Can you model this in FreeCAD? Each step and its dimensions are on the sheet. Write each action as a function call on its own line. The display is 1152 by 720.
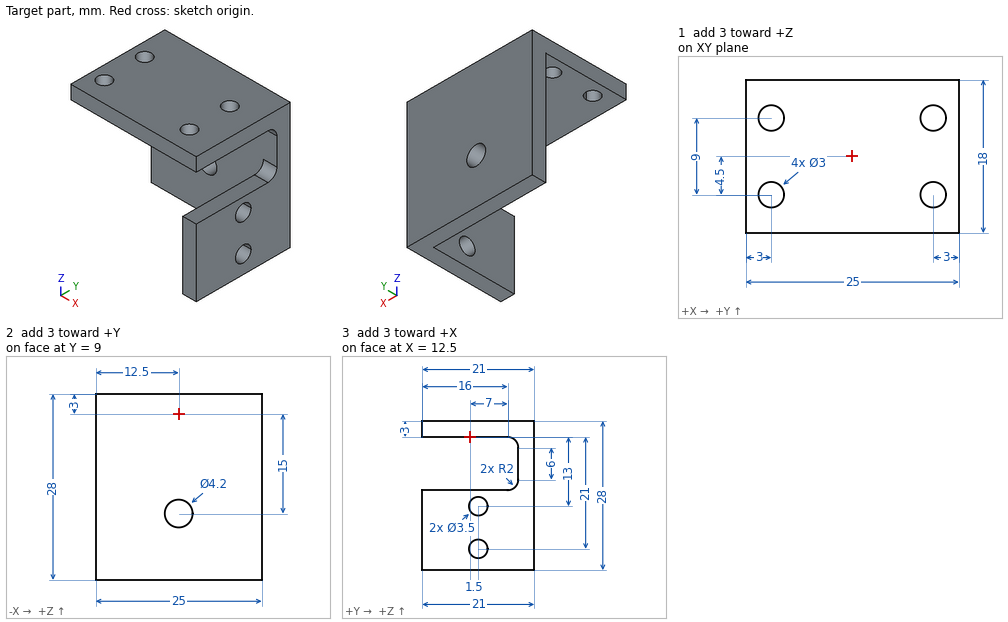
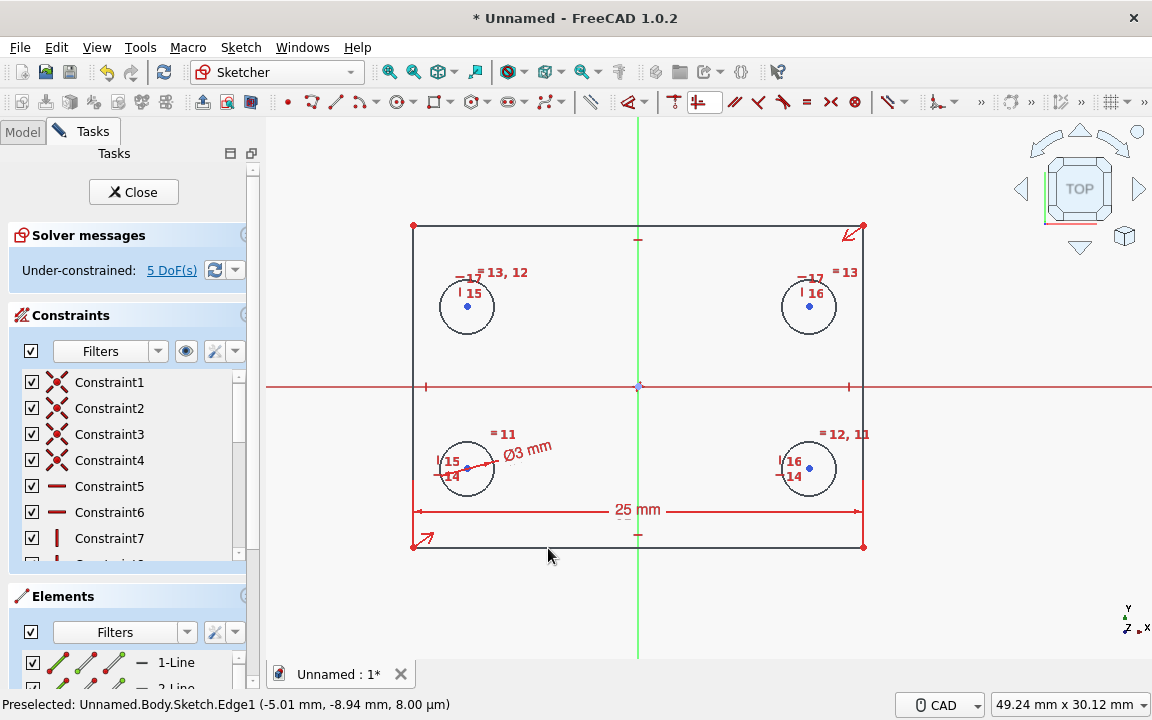
click(863, 451)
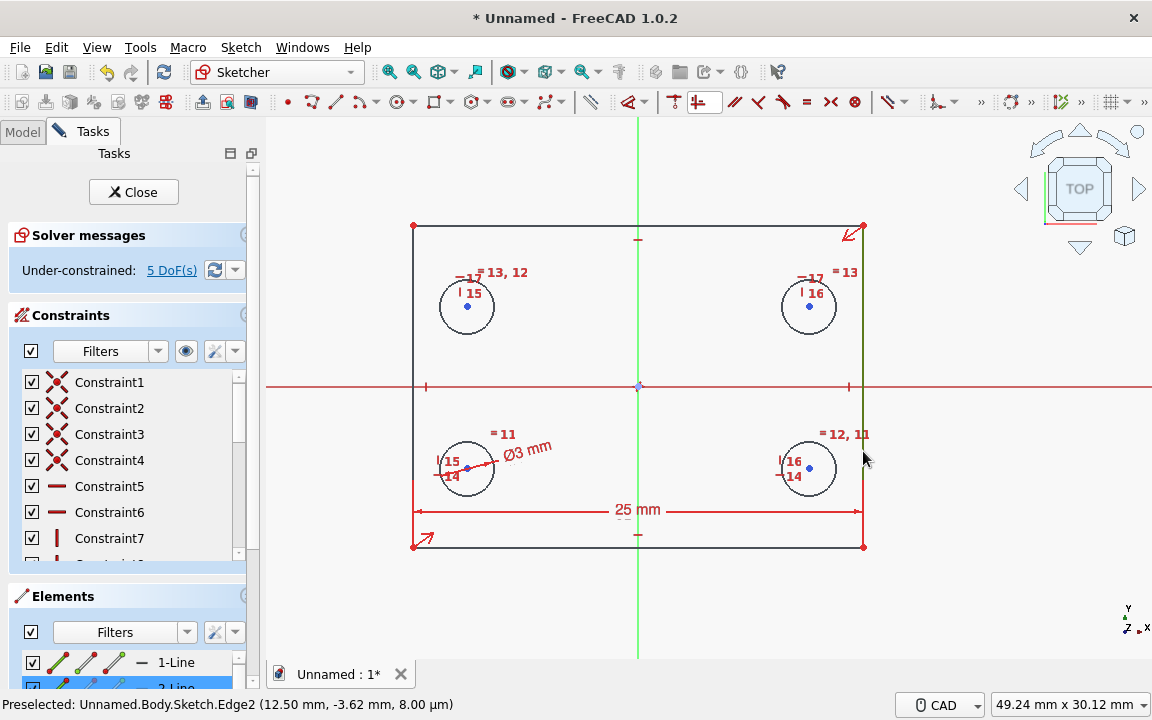
key(i)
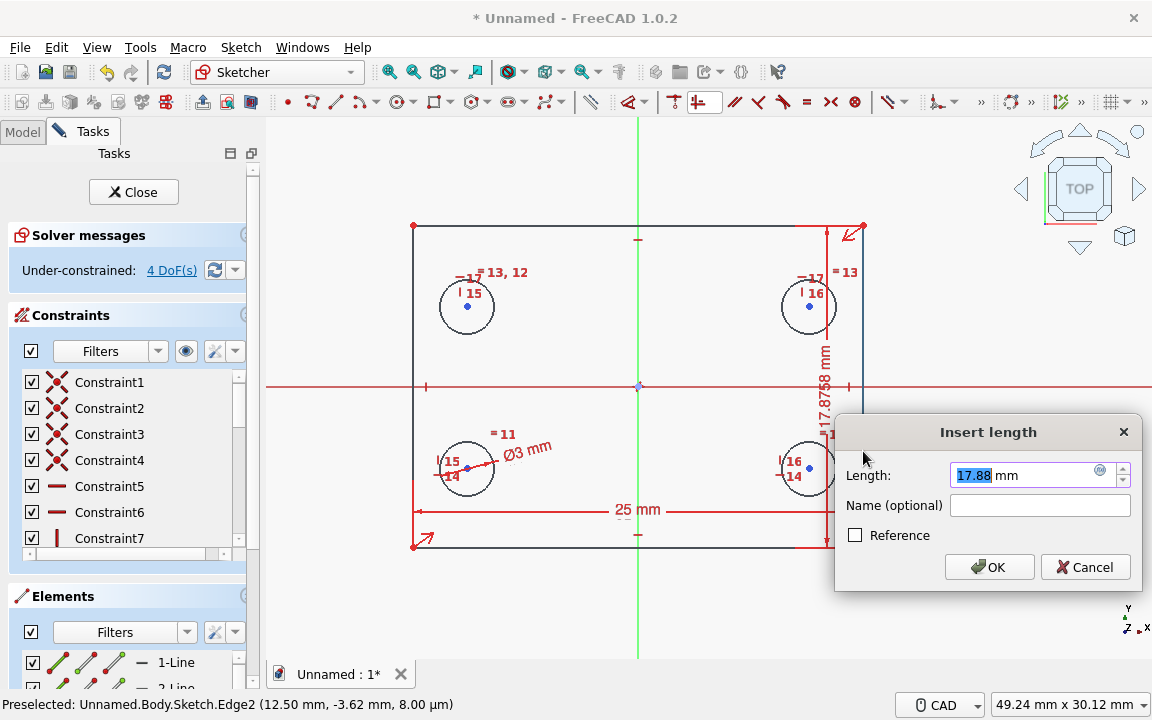
text(18)
key(Return)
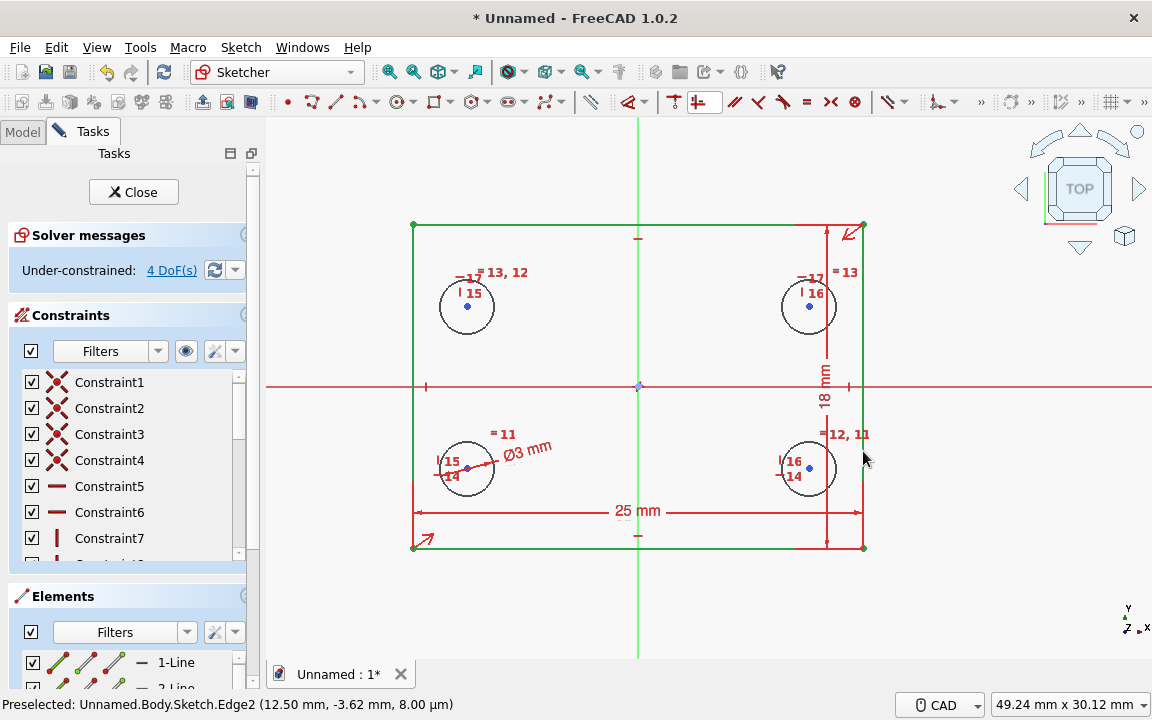
click(413, 549)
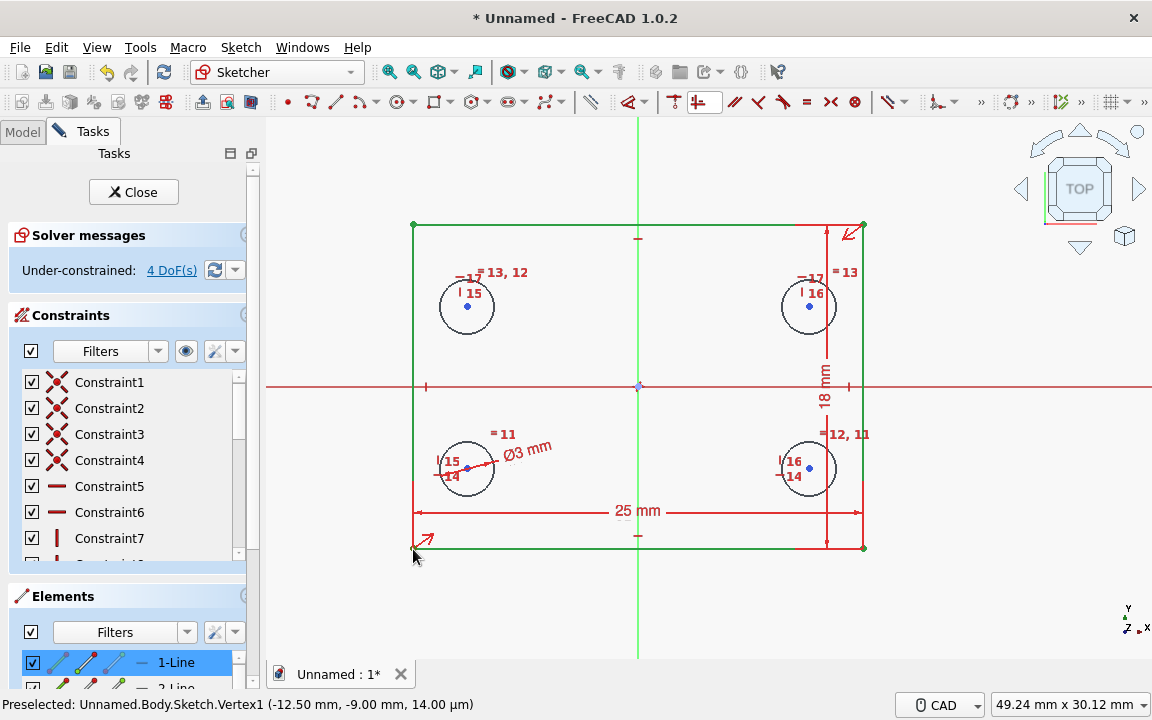
click(467, 469)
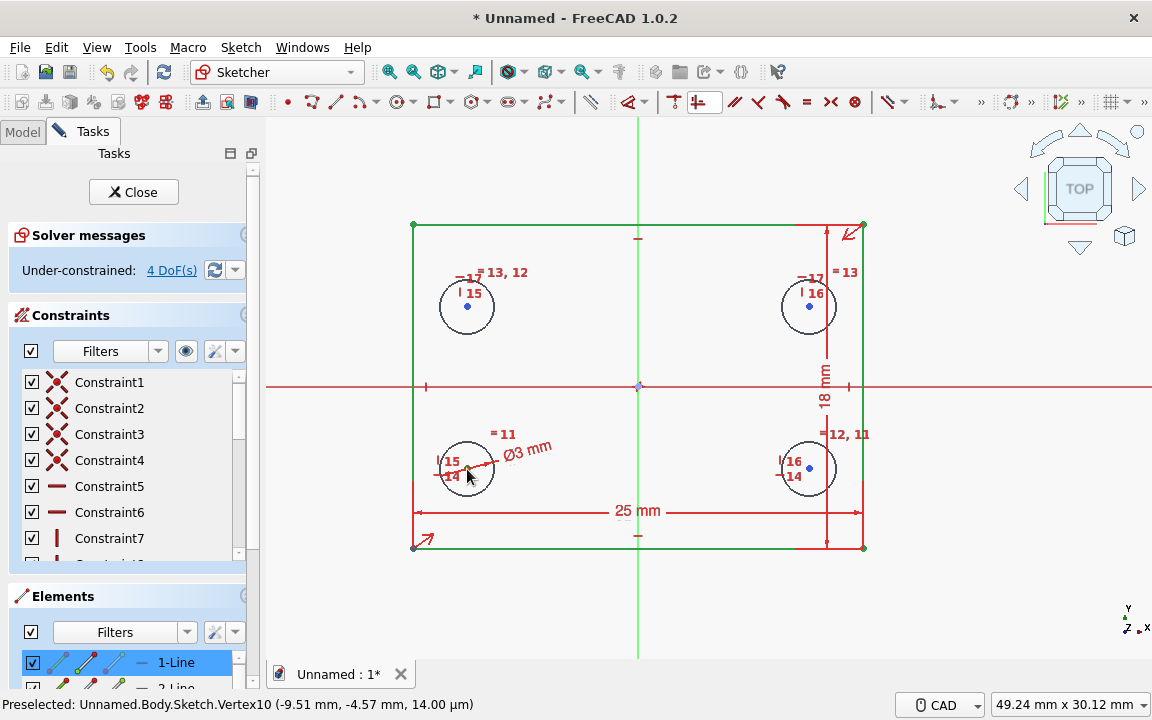
key(l)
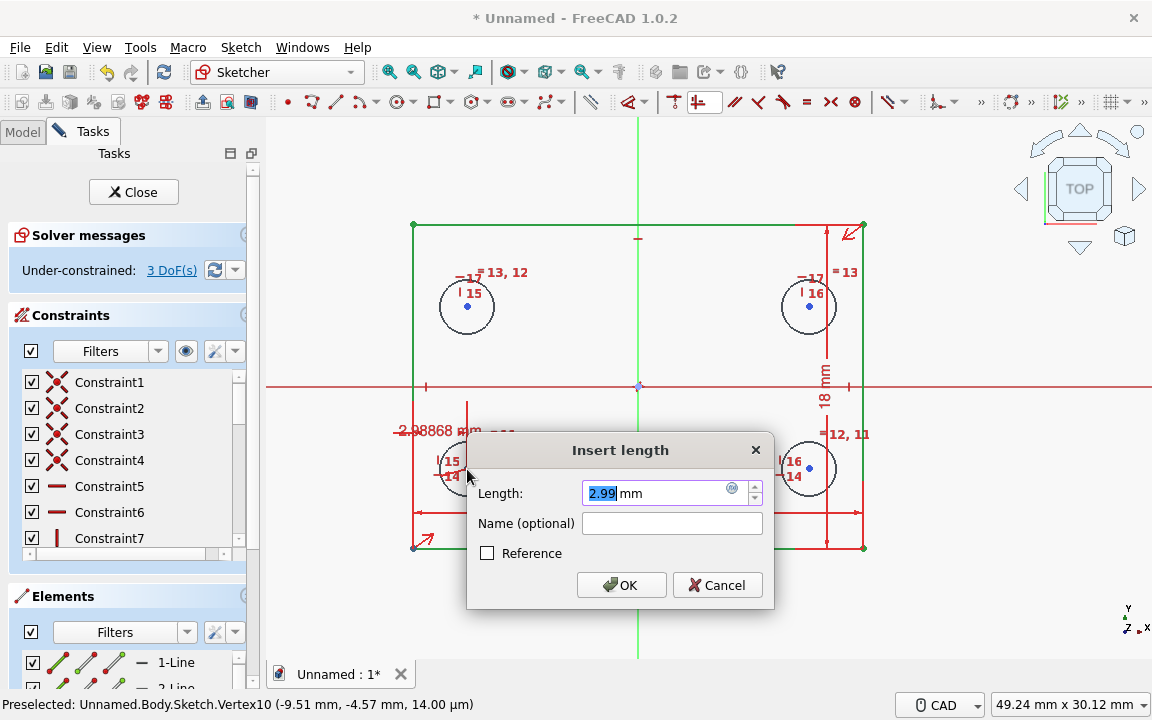
text(3)
key(Return)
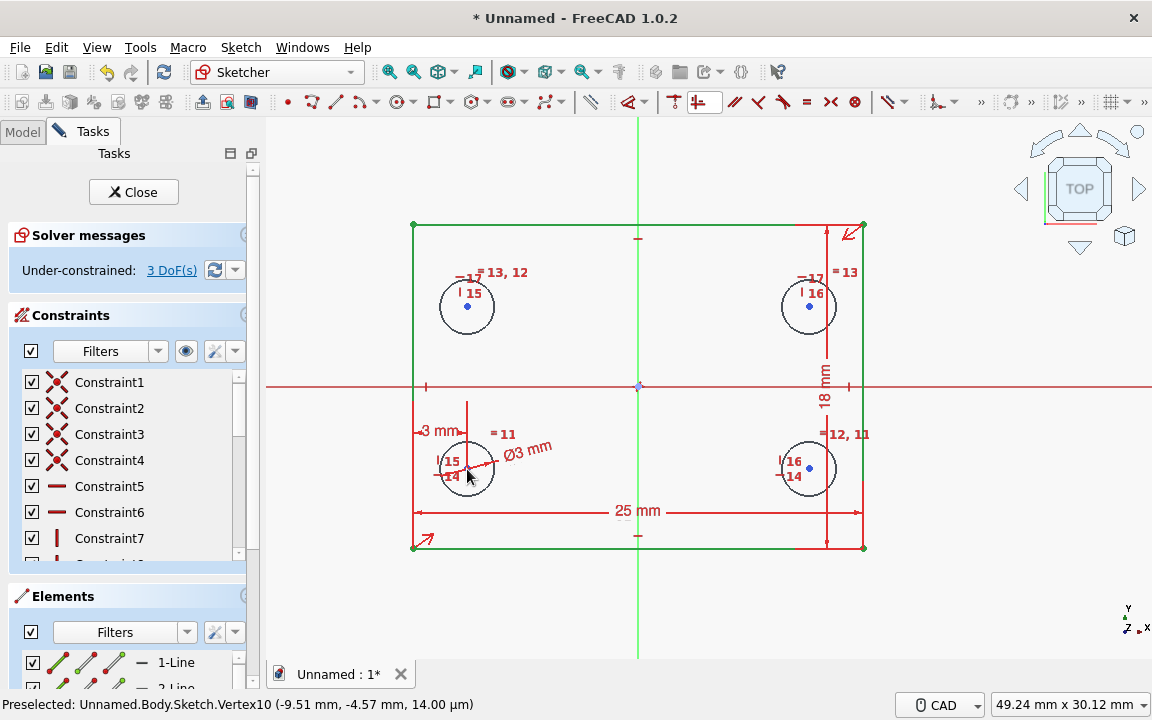
click(863, 549)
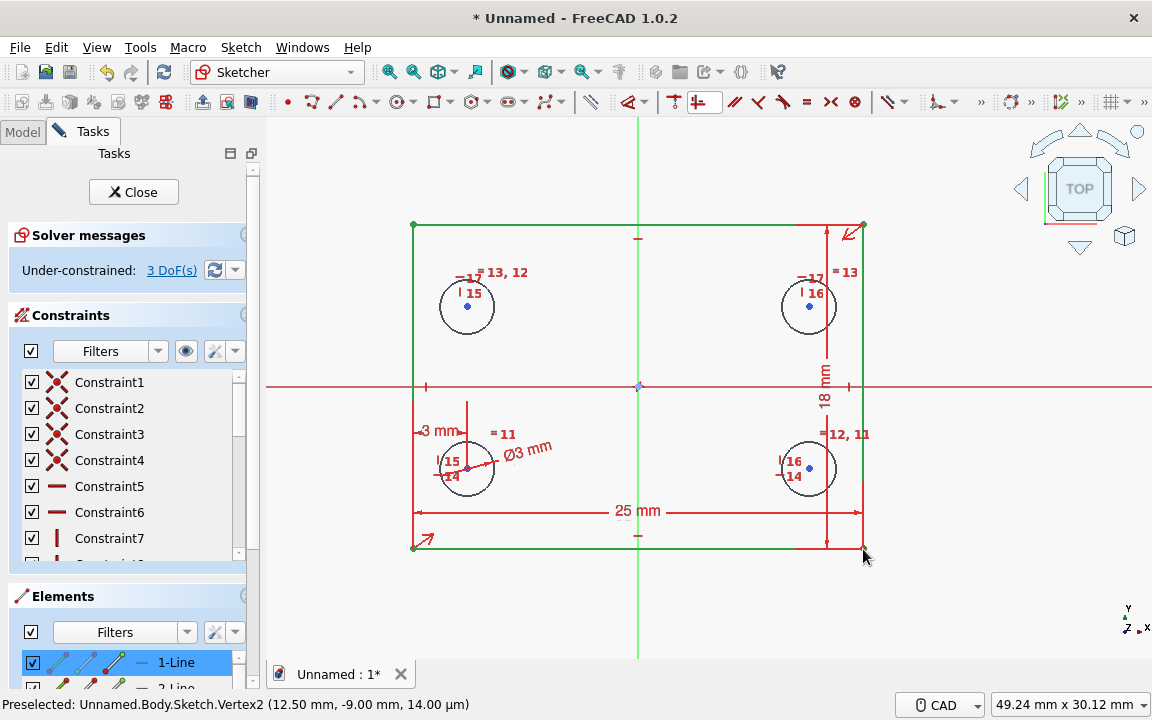
click(809, 469)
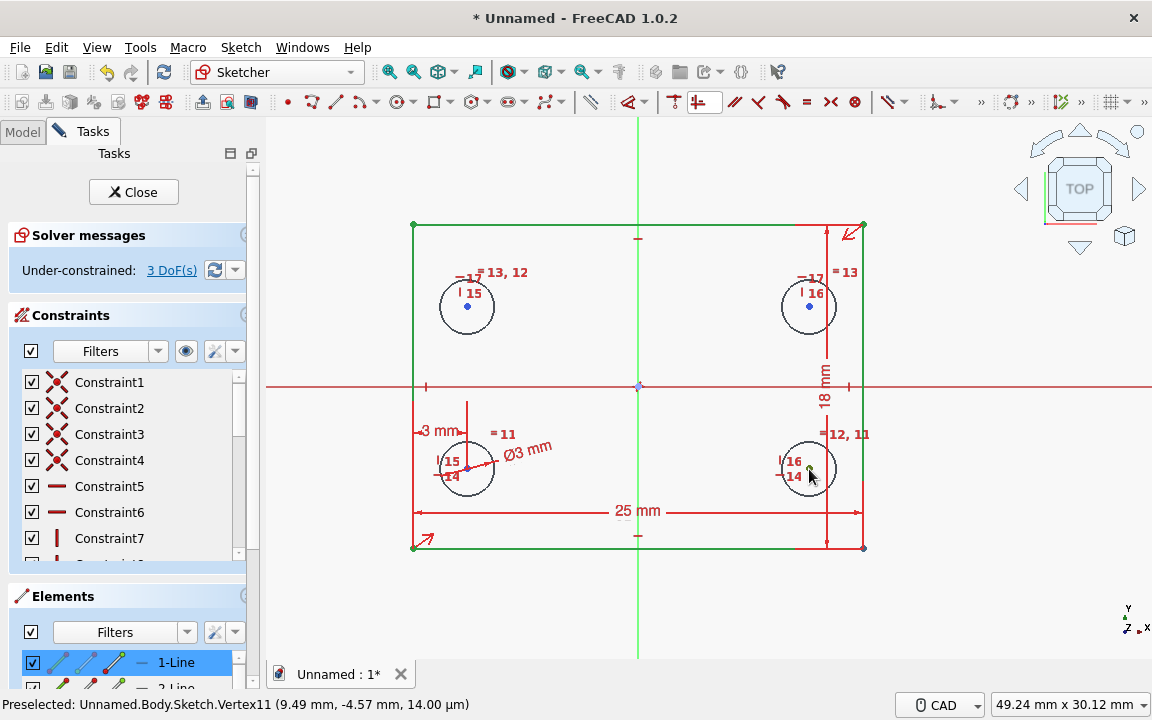
click(646, 102)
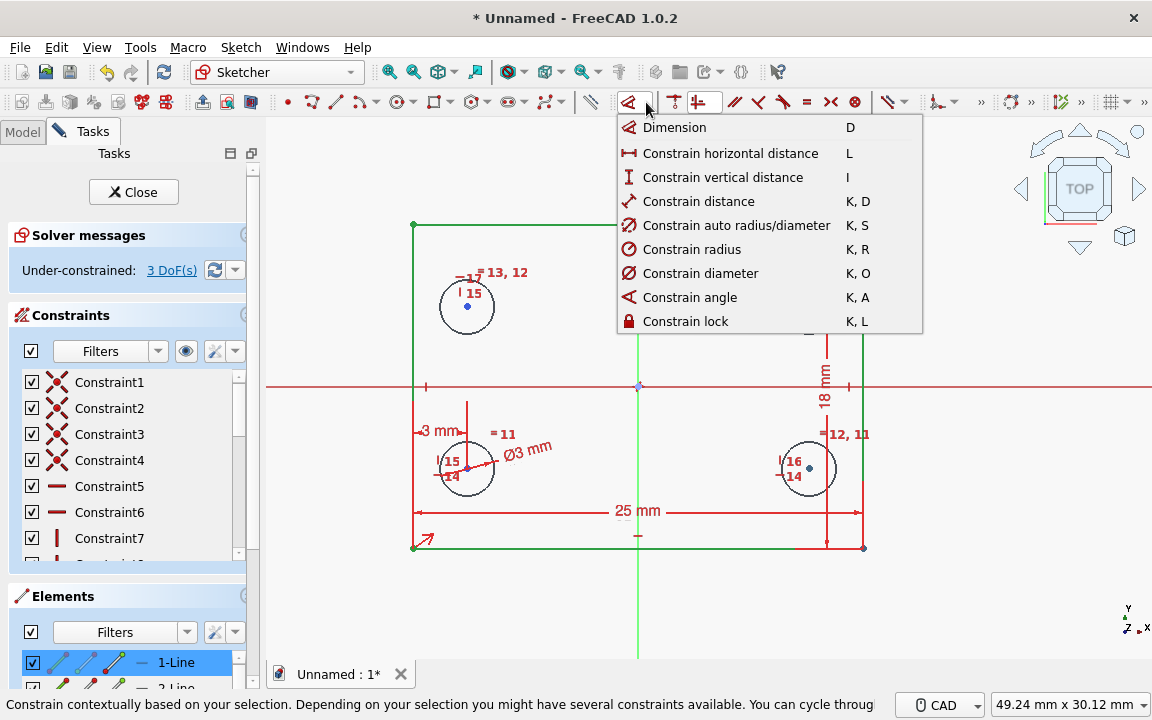
click(770, 153)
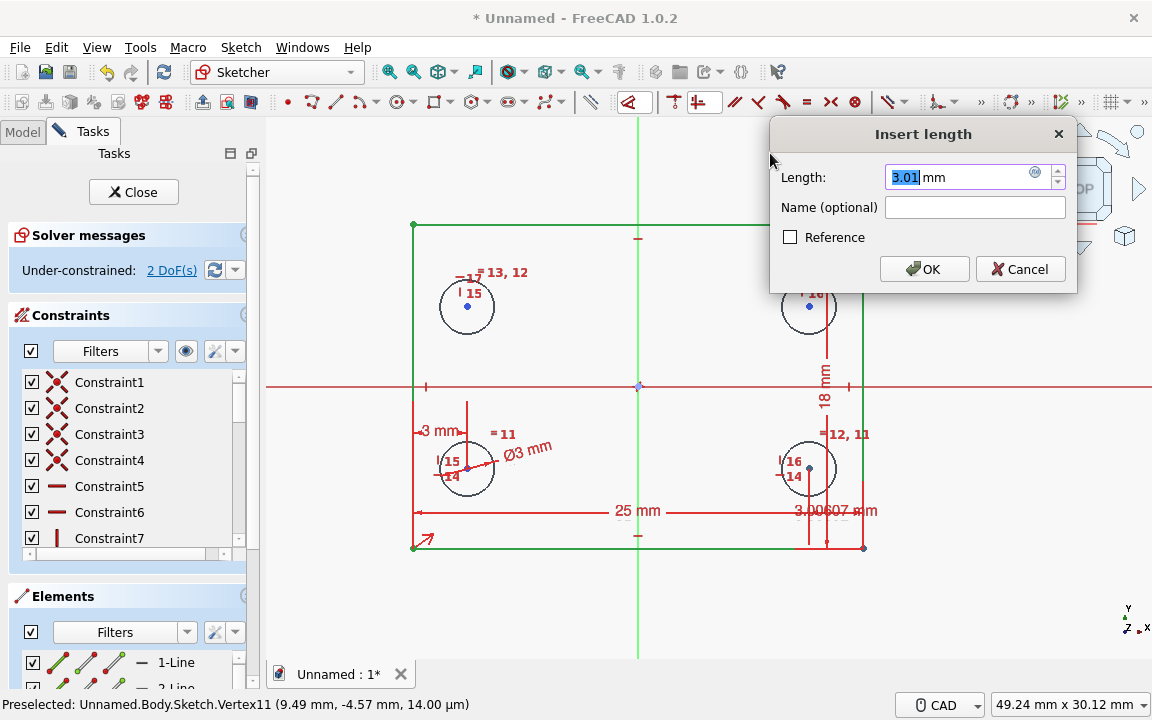
text(3)
key(Return)